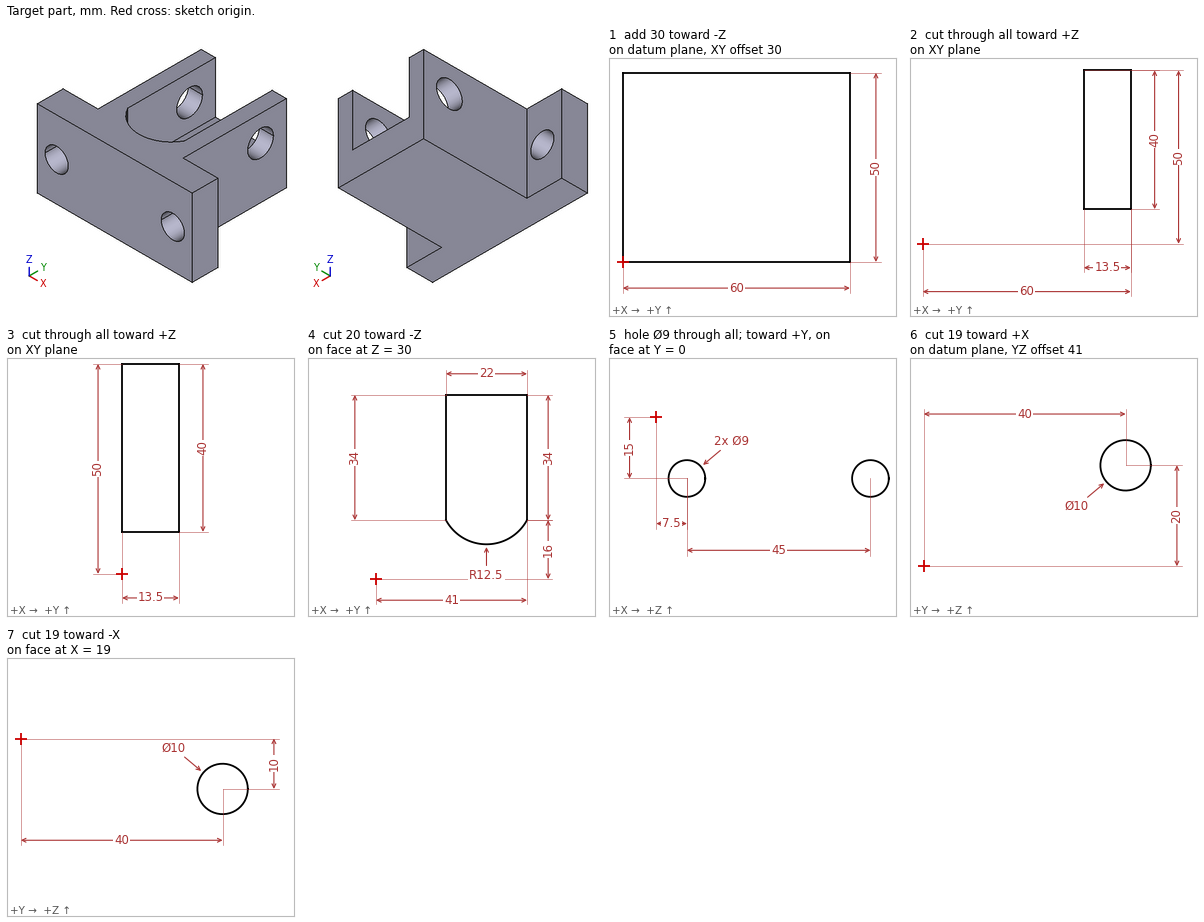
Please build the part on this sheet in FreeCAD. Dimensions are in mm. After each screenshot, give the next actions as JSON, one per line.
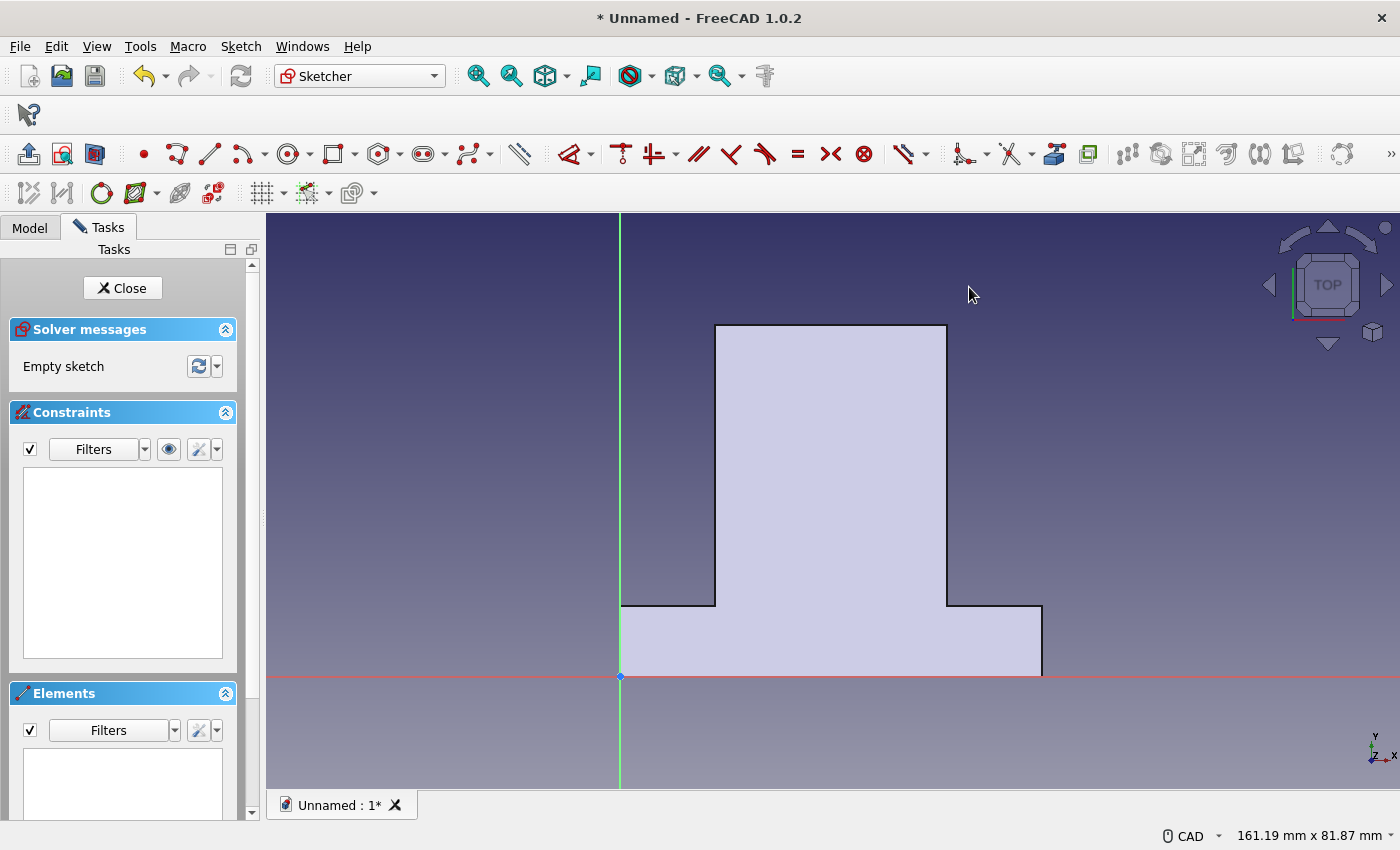
{"action": "key", "text": "g m"}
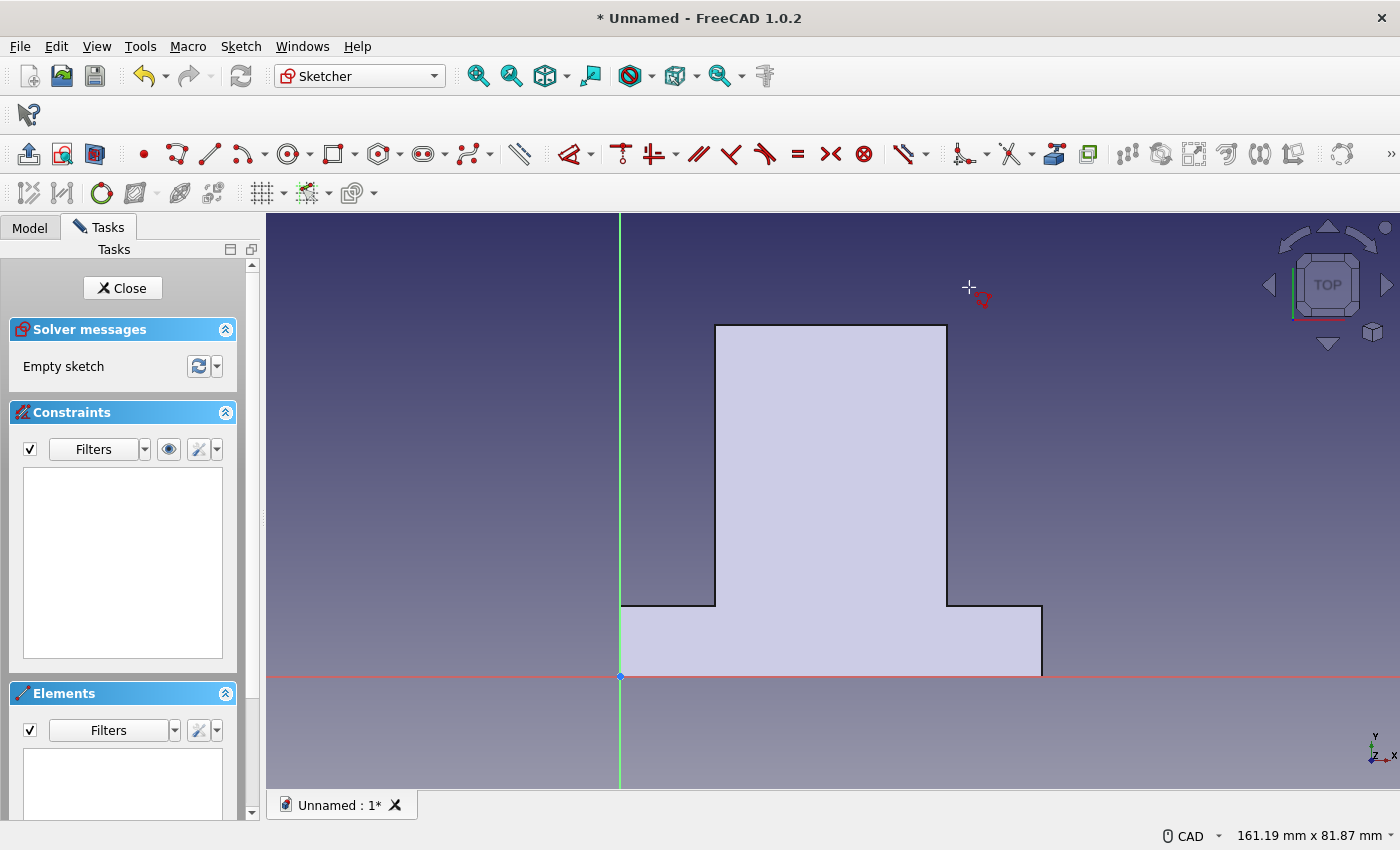
{"action": "left_click", "coordinate": [909, 564]}
{"action": "left_click", "coordinate": [909, 325]}
{"action": "left_click", "coordinate": [754, 325]}
{"action": "left_click", "coordinate": [754, 564]}
{"action": "right_click", "coordinate": [754, 564]}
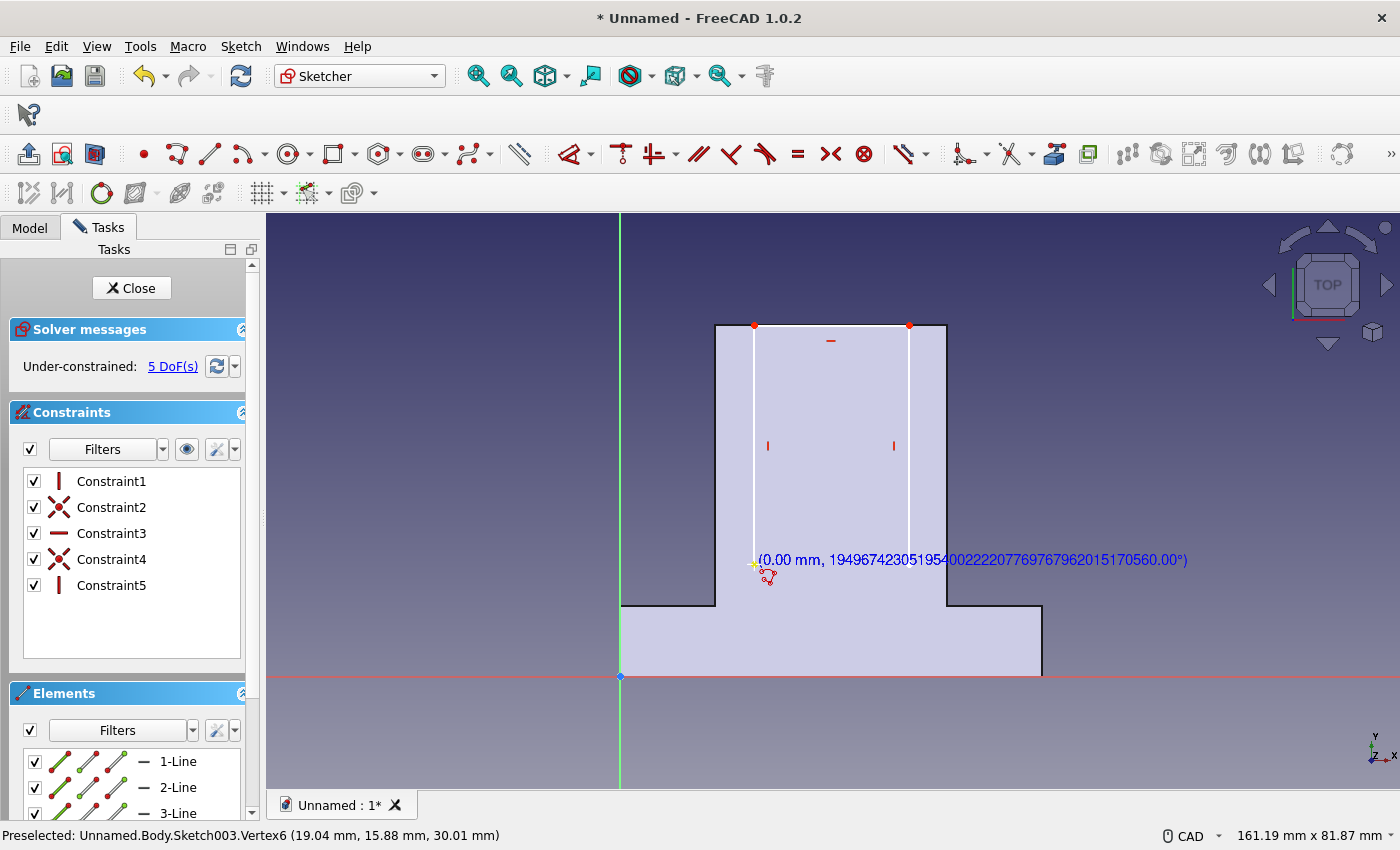
{"action": "key", "text": "g 3 a"}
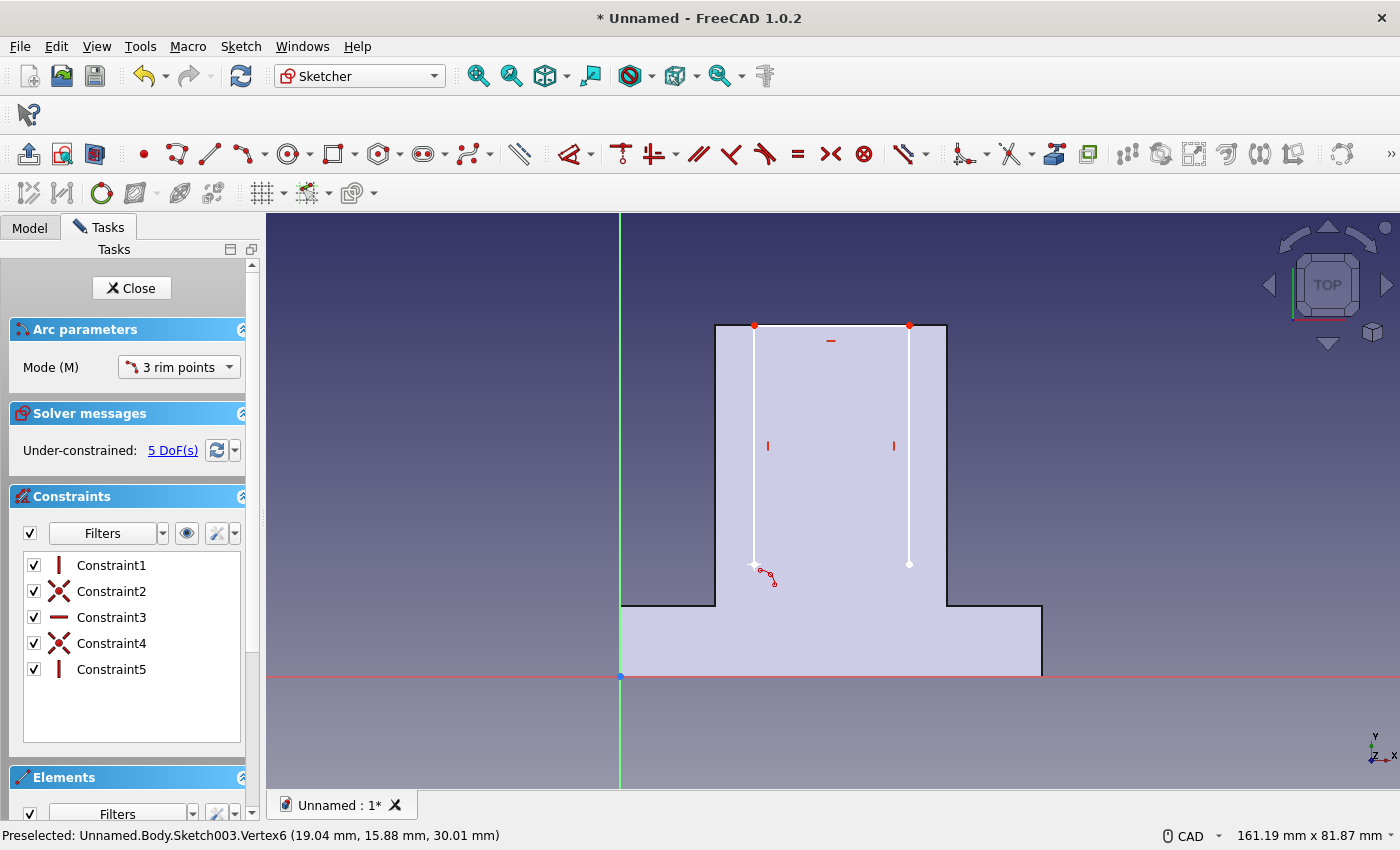
{"action": "left_click", "coordinate": [754, 565]}
{"action": "left_click", "coordinate": [909, 565]}
{"action": "left_click", "coordinate": [831, 610]}
{"action": "key", "text": "Escape"}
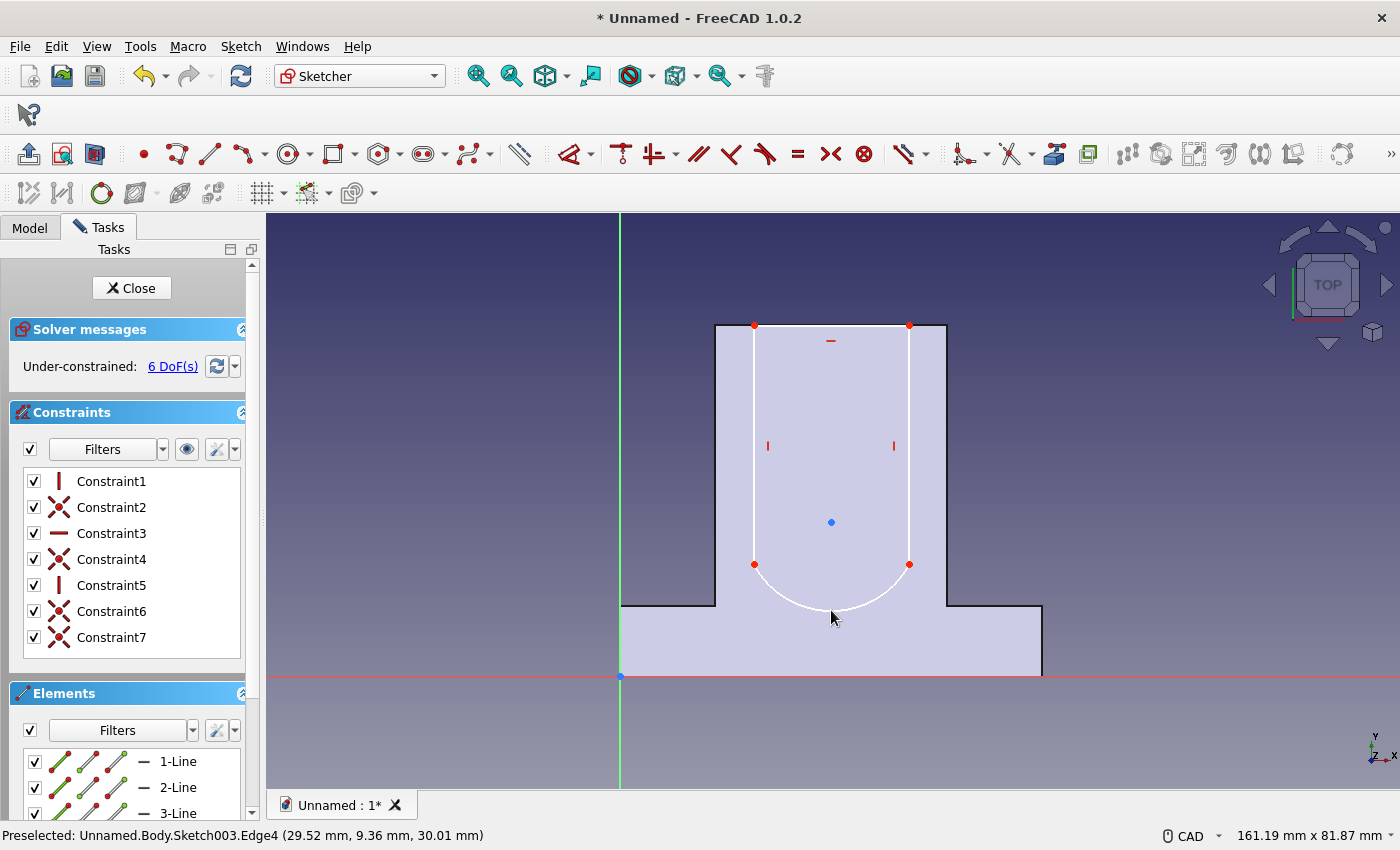
{"action": "left_click", "coordinate": [795, 603]}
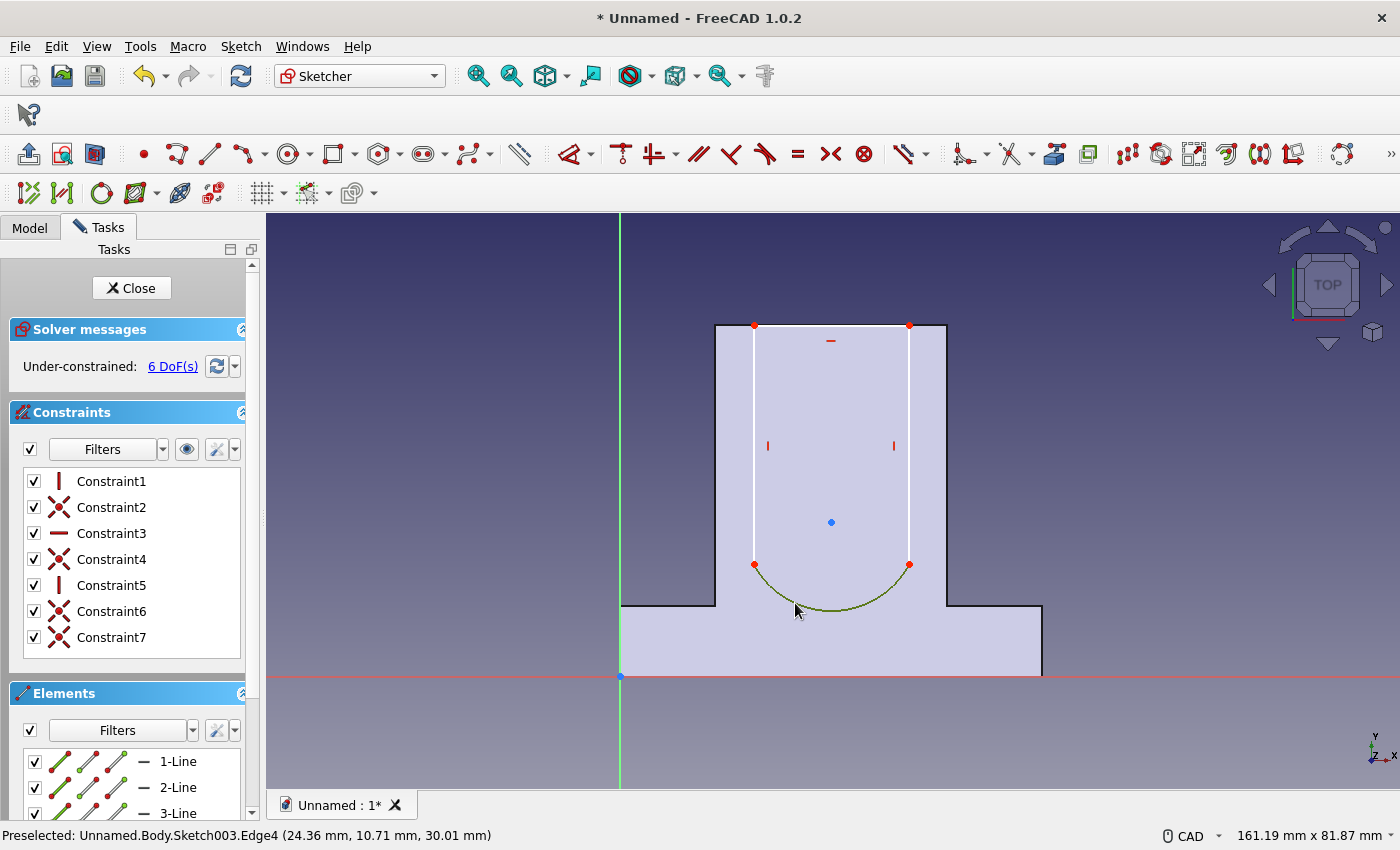
{"action": "key", "text": "k r"}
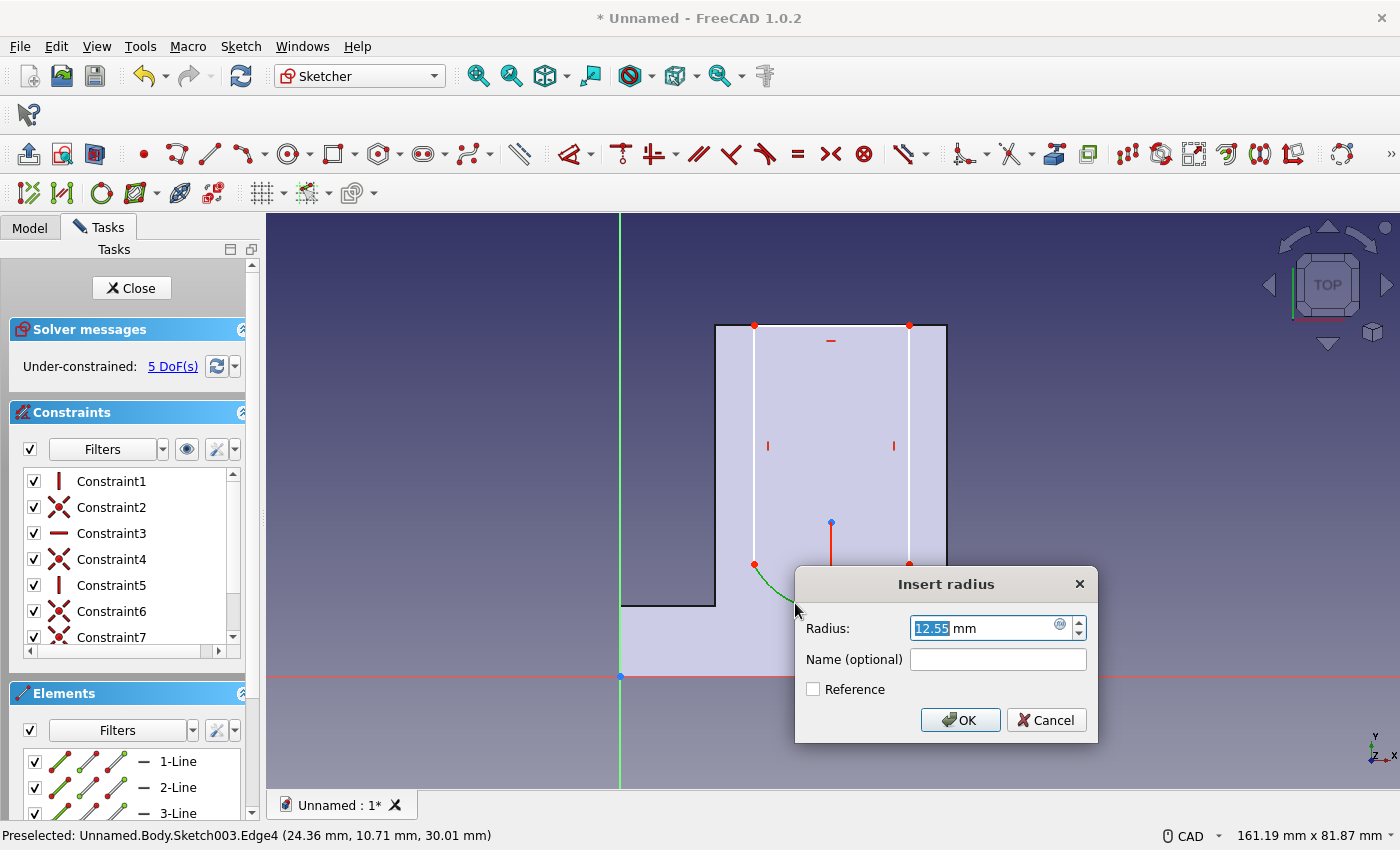
{"action": "type", "text": "12.5"}
{"action": "key", "text": "Return"}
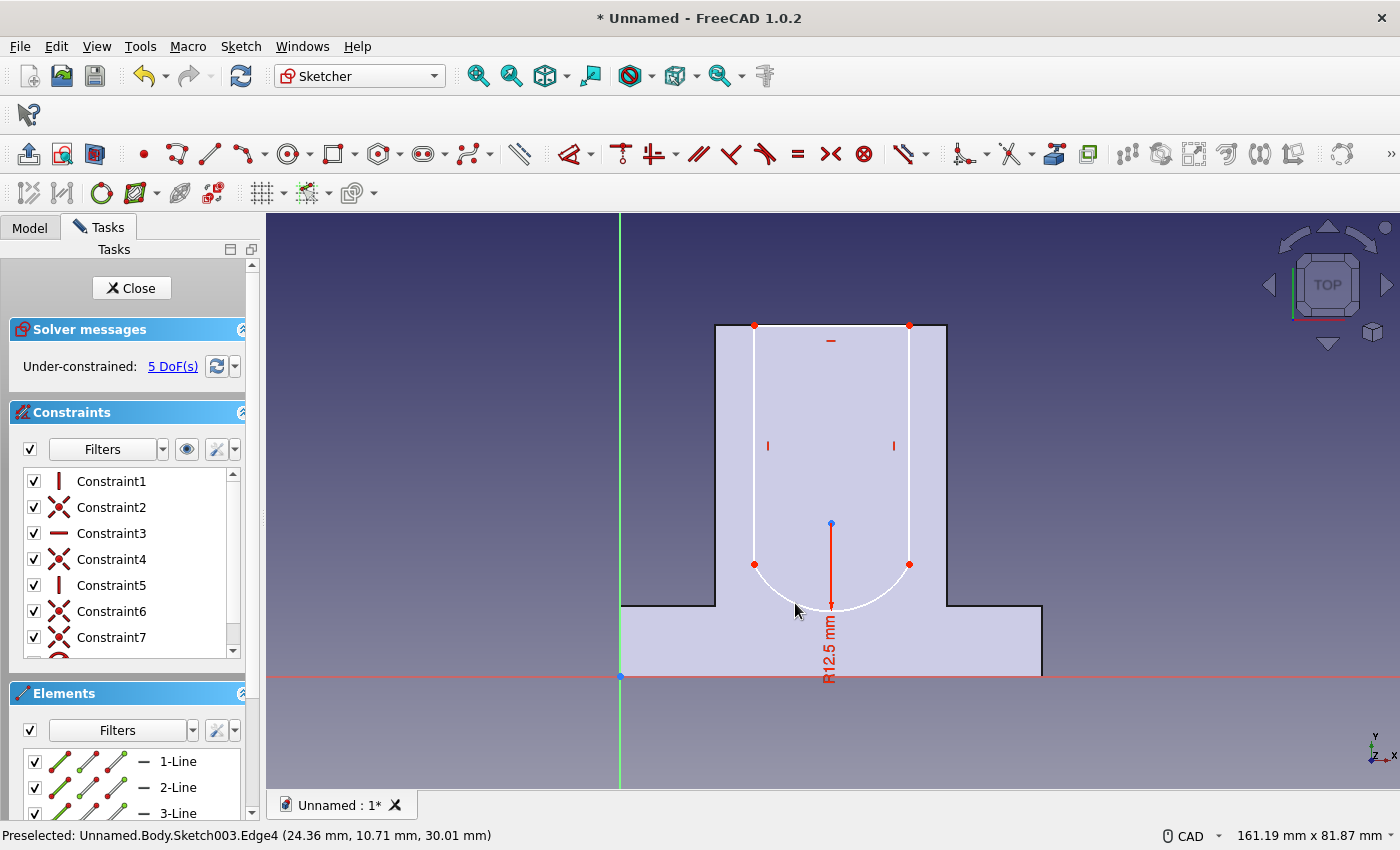
{"action": "left_click", "coordinate": [909, 493]}